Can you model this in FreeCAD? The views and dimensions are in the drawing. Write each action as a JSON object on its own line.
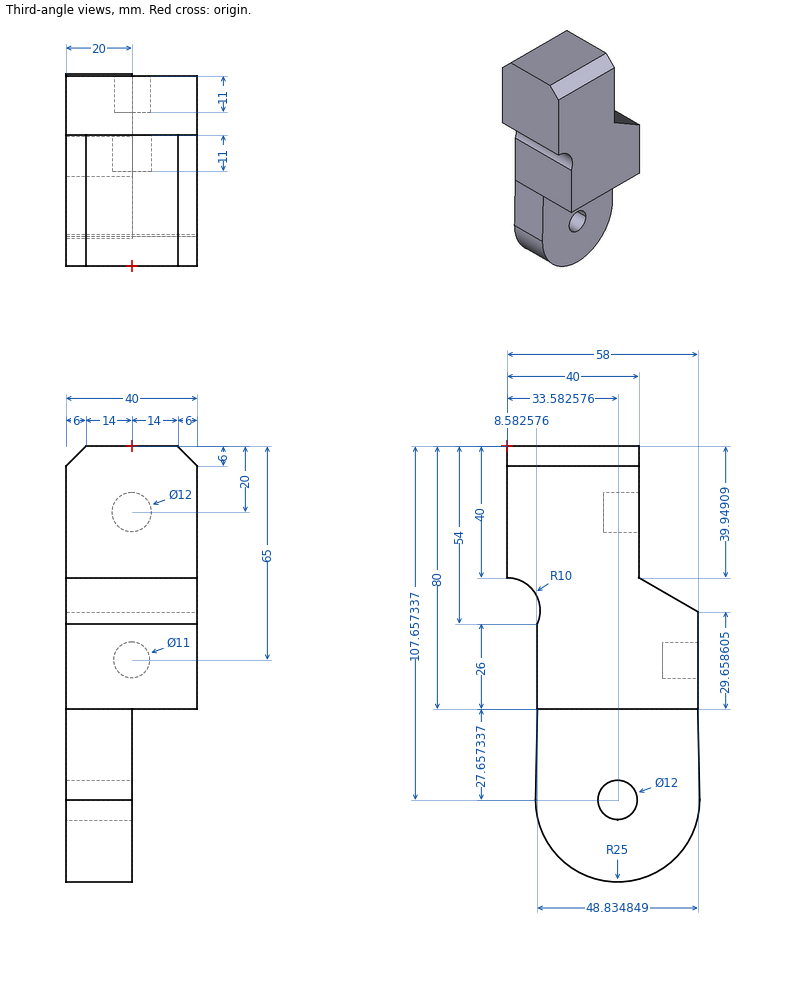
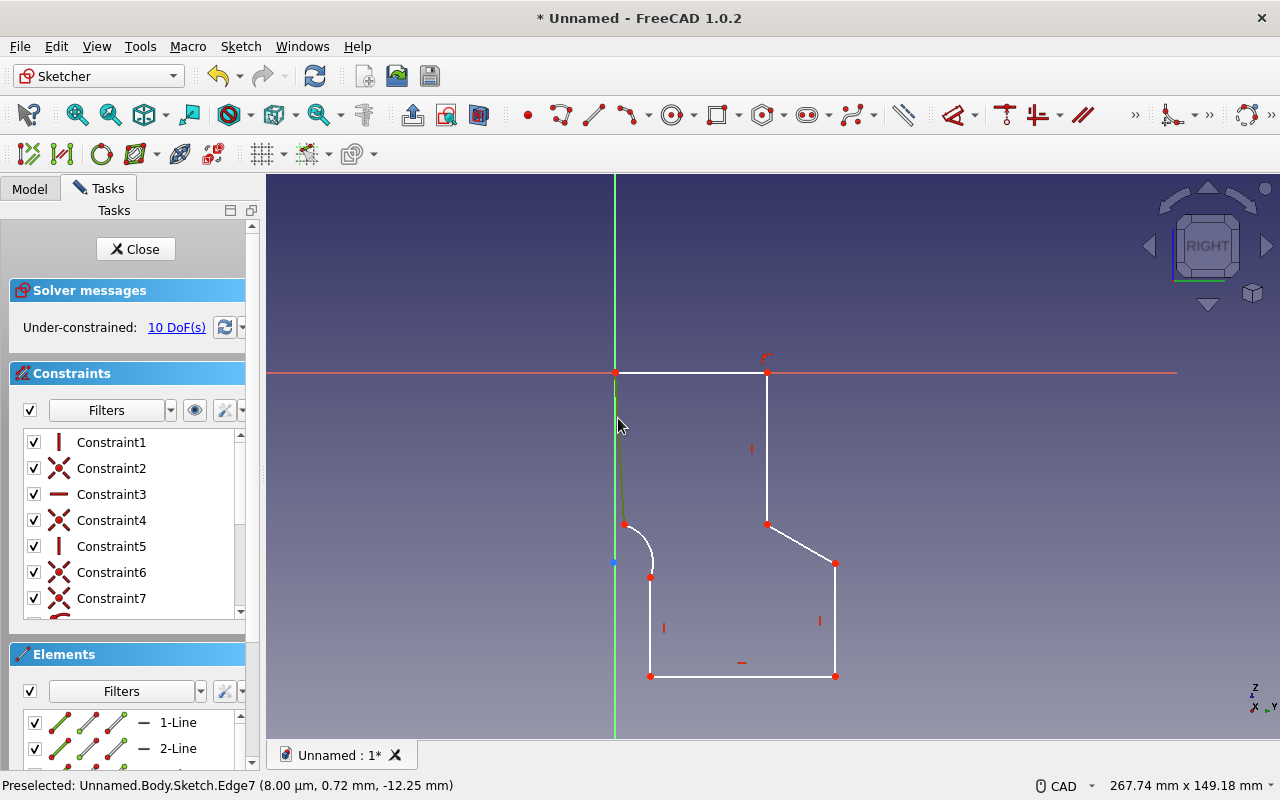
{"action": "key", "text": "v"}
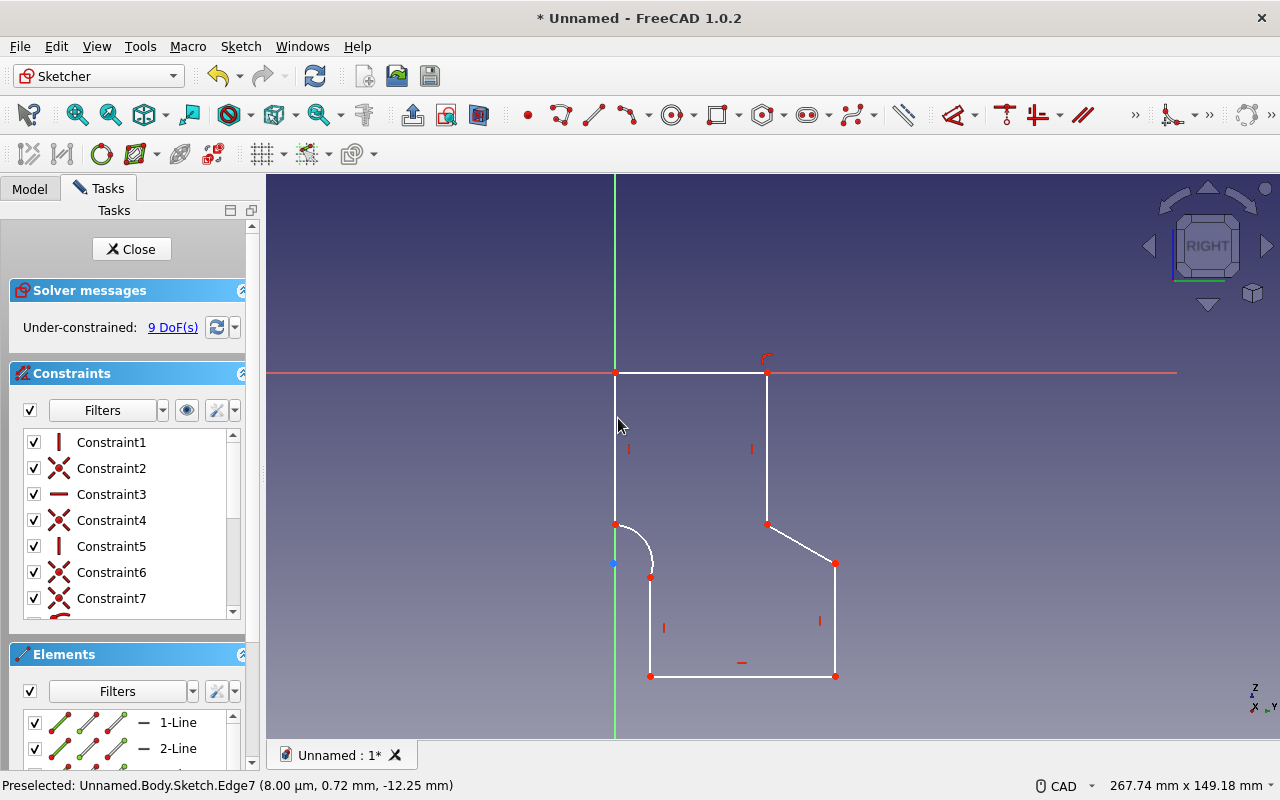
{"action": "left_click", "coordinate": [614, 564]}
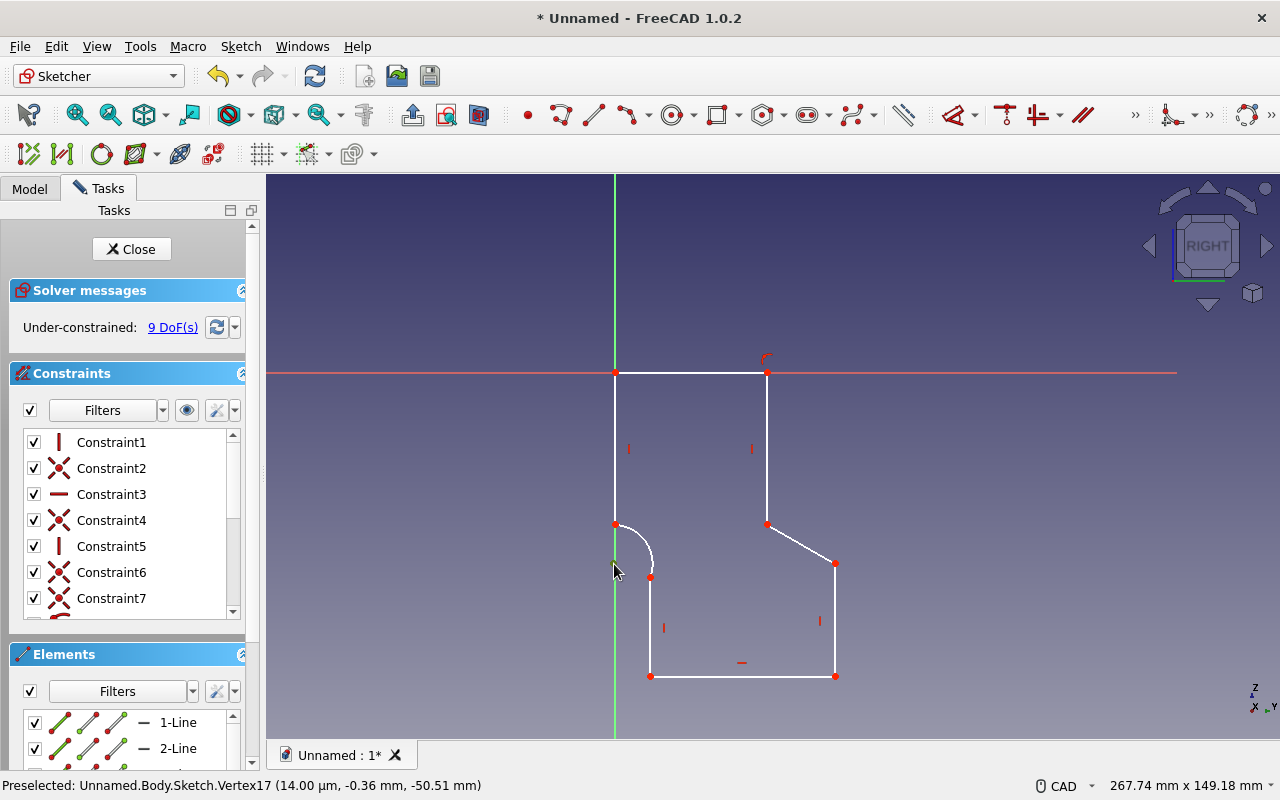
{"action": "left_click", "coordinate": [615, 675]}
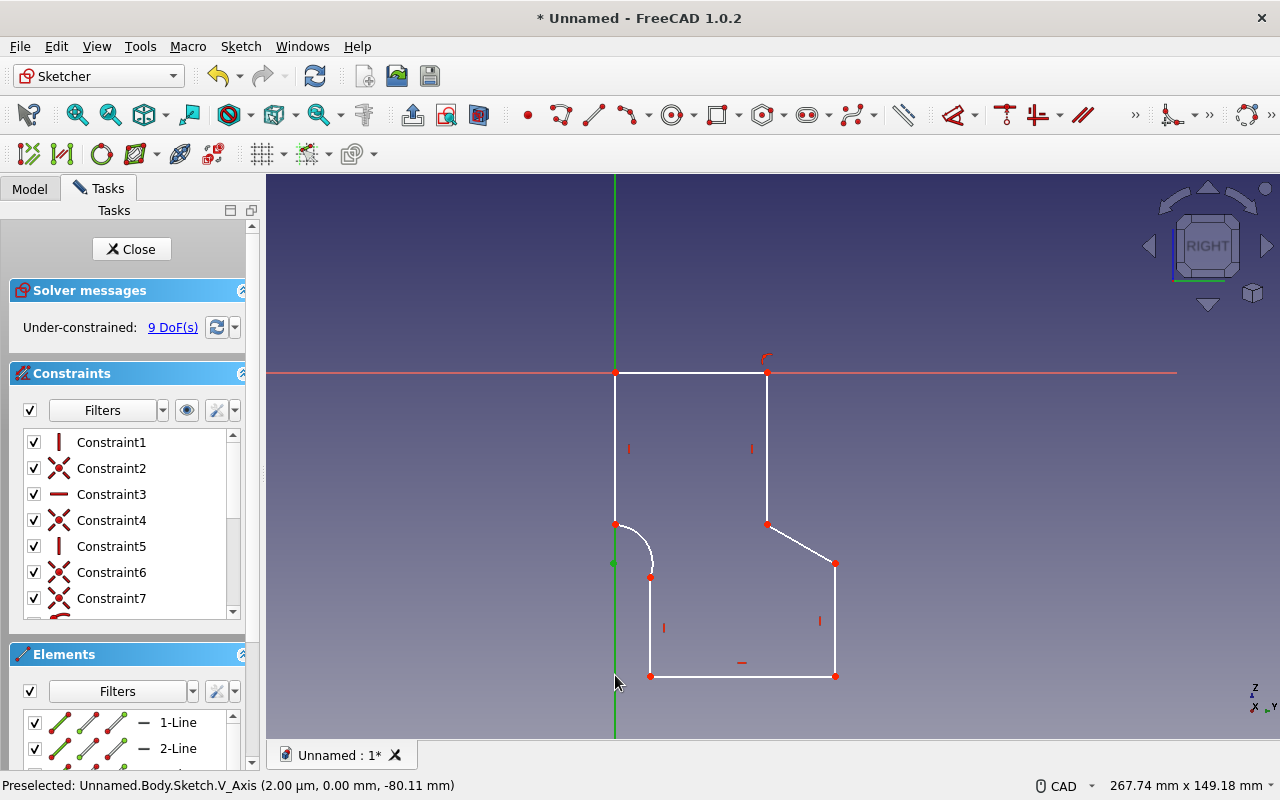
{"action": "left_click", "coordinate": [1005, 116]}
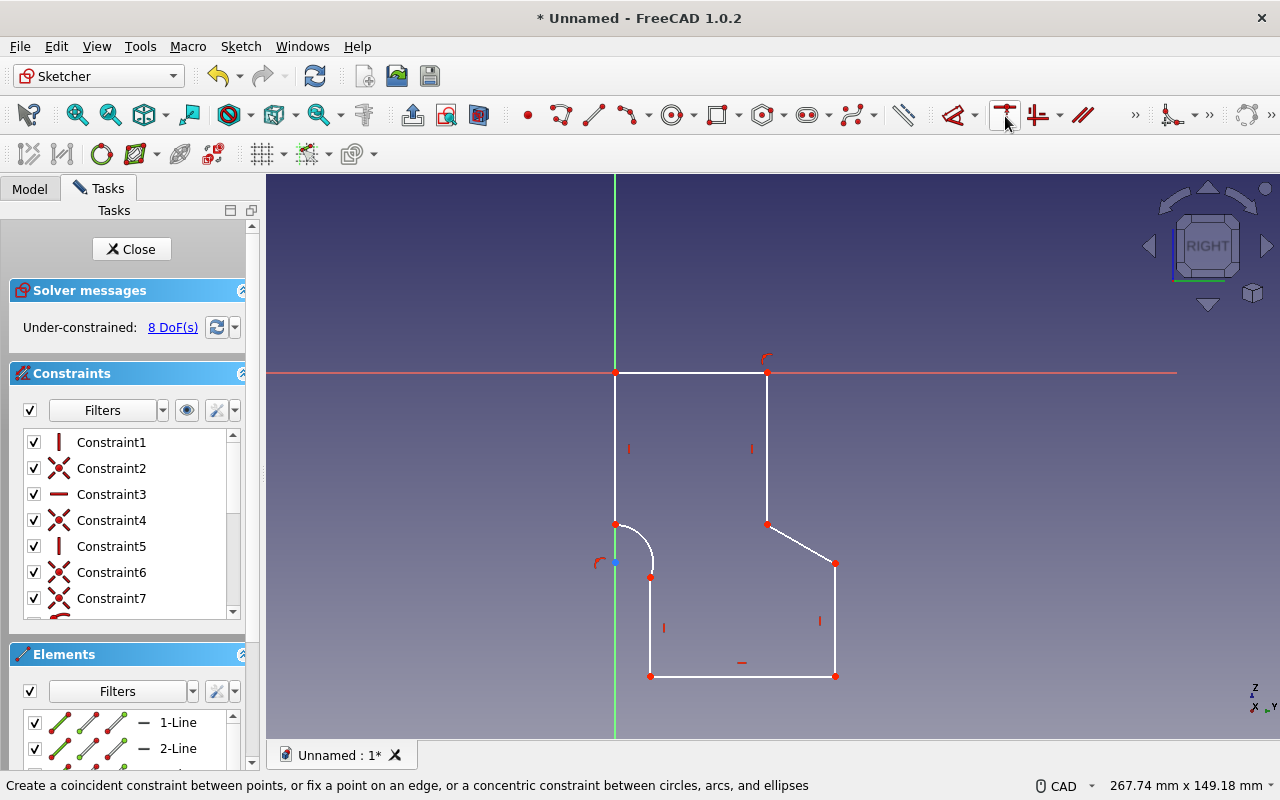
{"action": "left_click", "coordinate": [652, 556]}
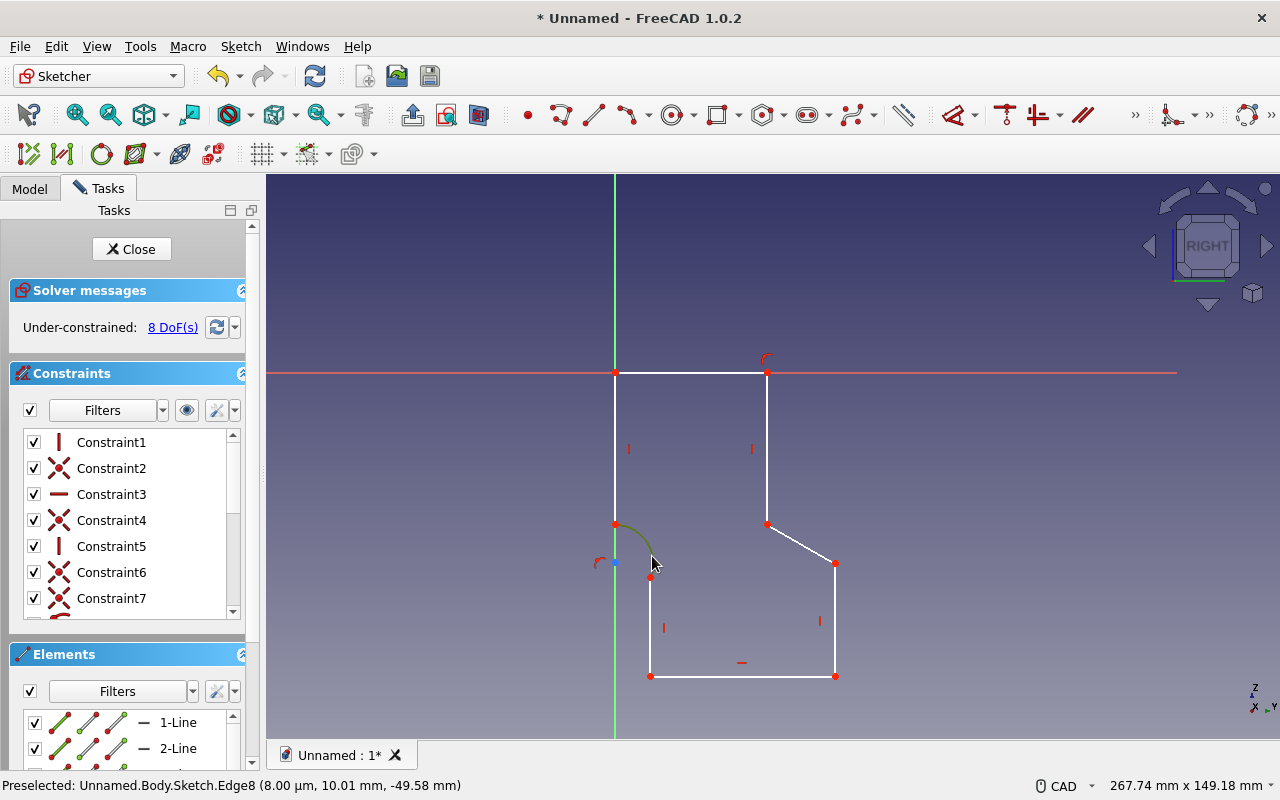
{"action": "key", "text": "k r"}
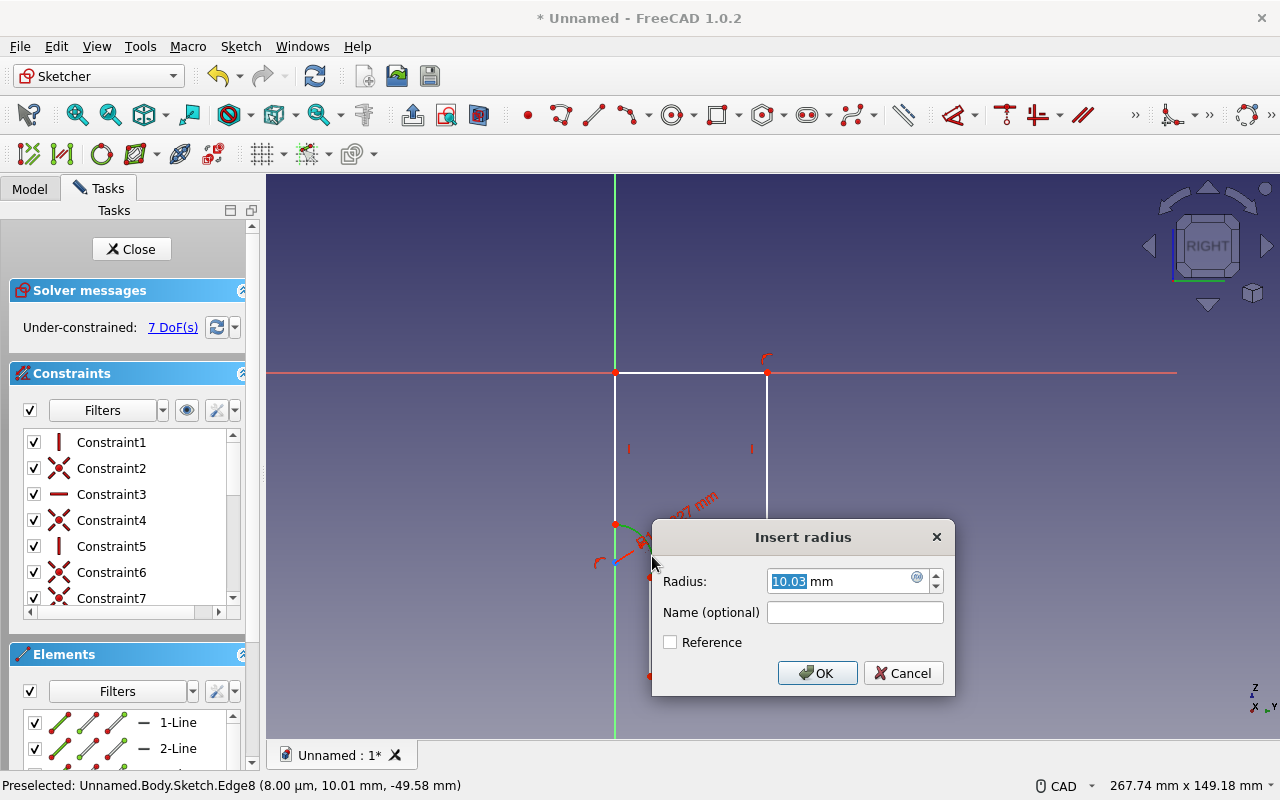
{"action": "type", "text": "10"}
{"action": "key", "text": "Return"}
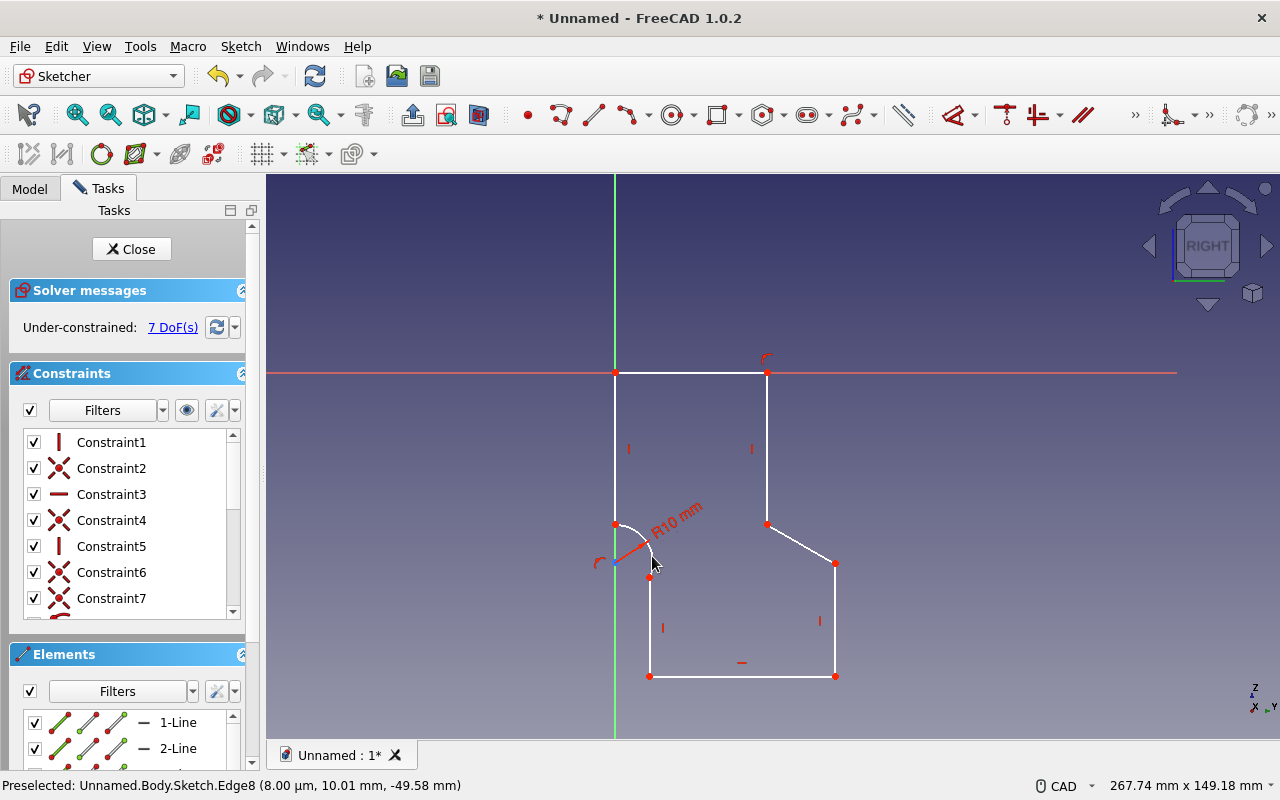
{"action": "left_click", "coordinate": [650, 608]}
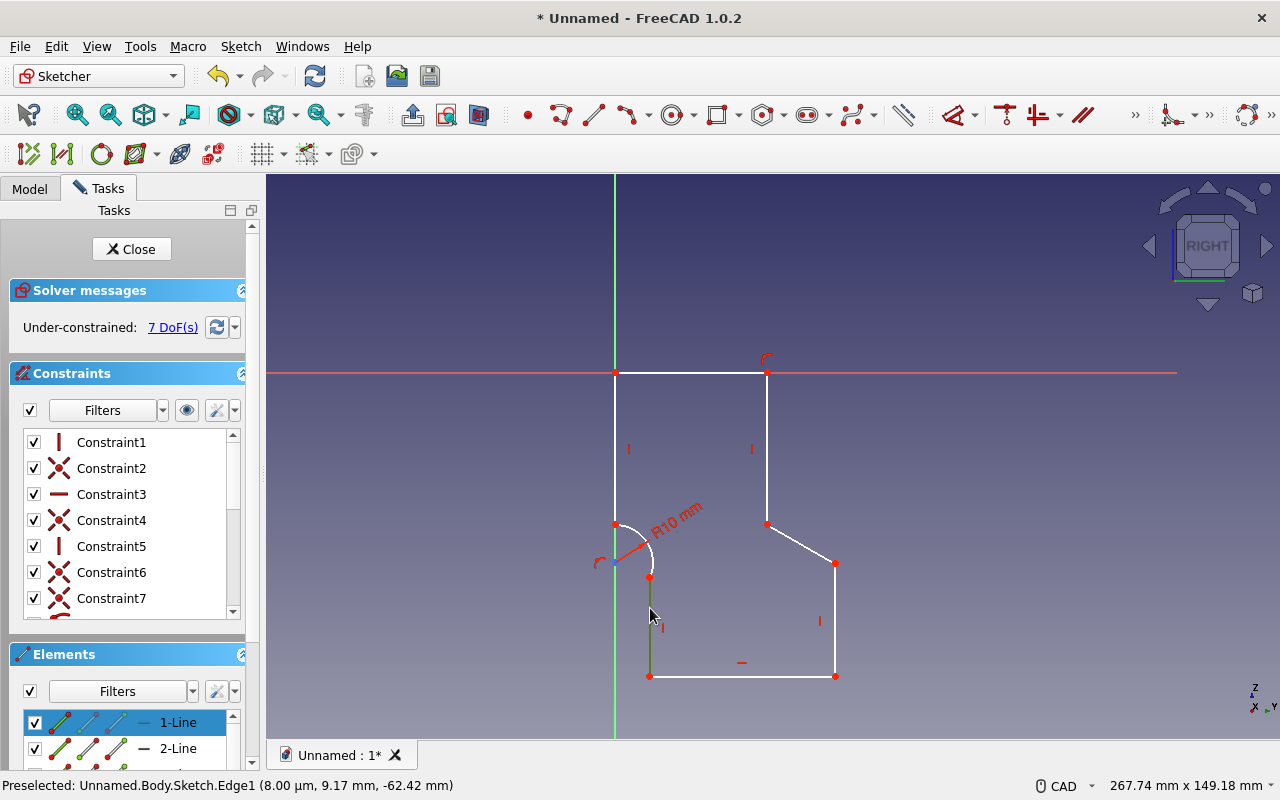
{"action": "left_click", "coordinate": [974, 116]}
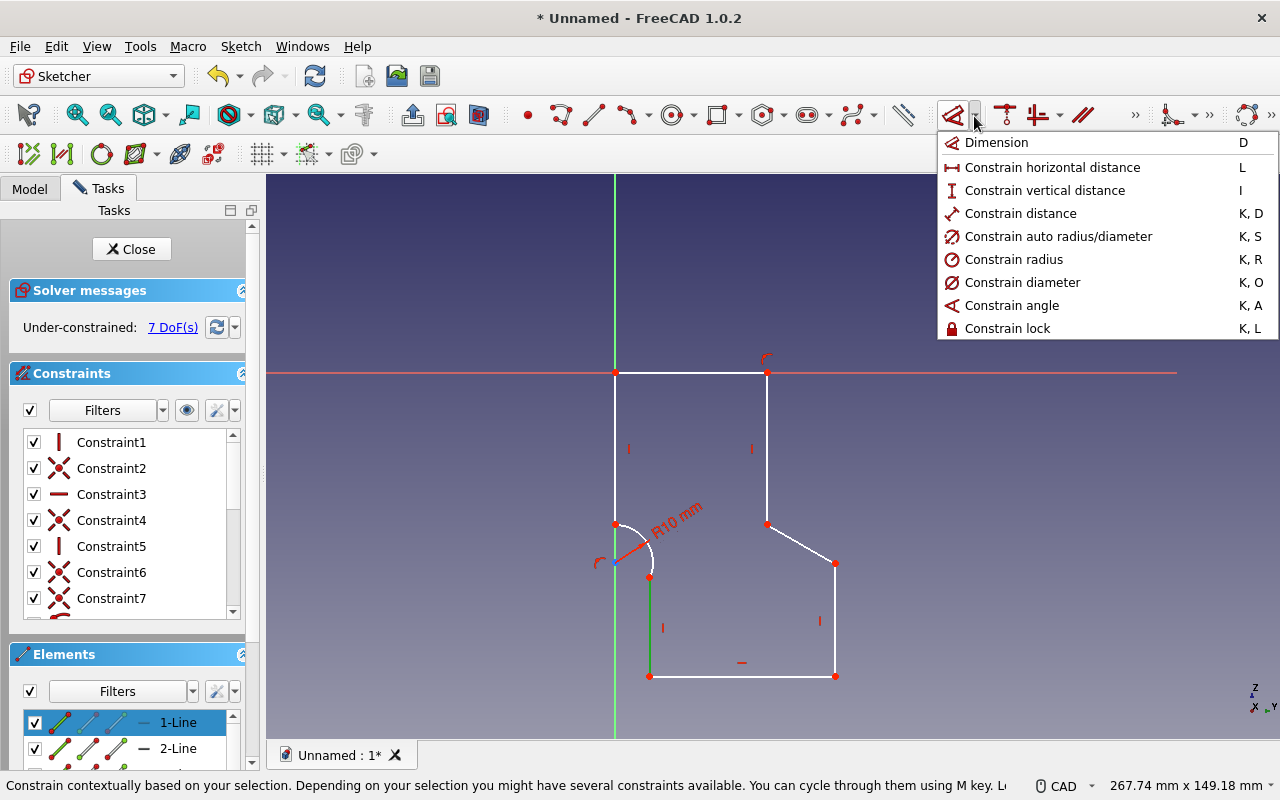
{"action": "left_click", "coordinate": [1108, 190]}